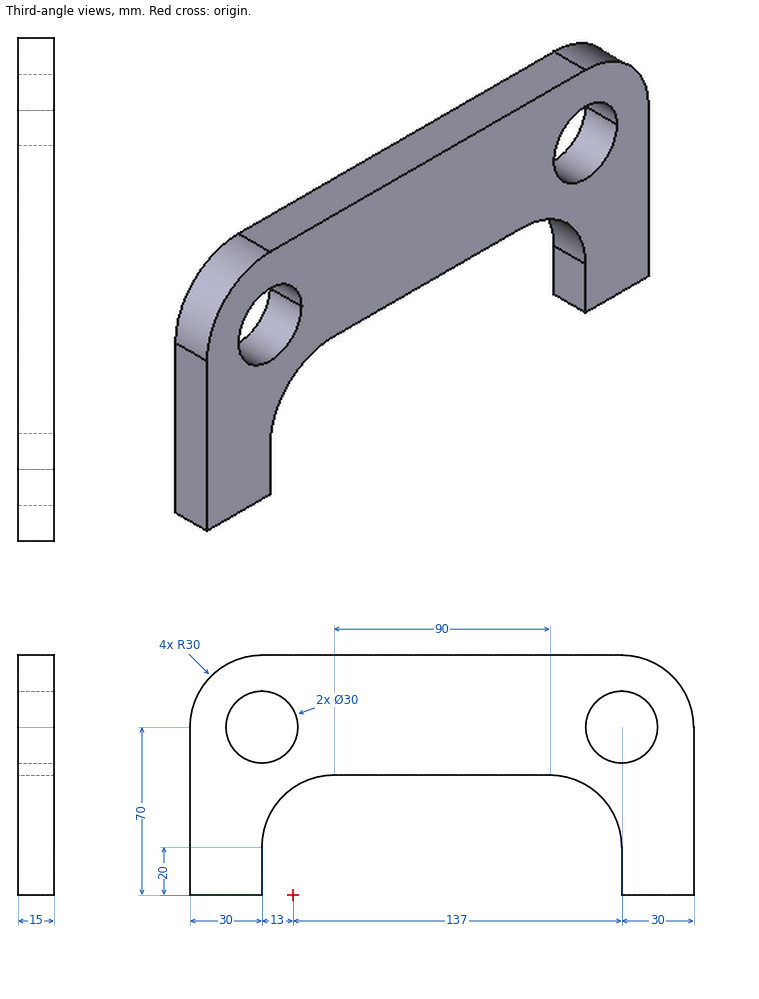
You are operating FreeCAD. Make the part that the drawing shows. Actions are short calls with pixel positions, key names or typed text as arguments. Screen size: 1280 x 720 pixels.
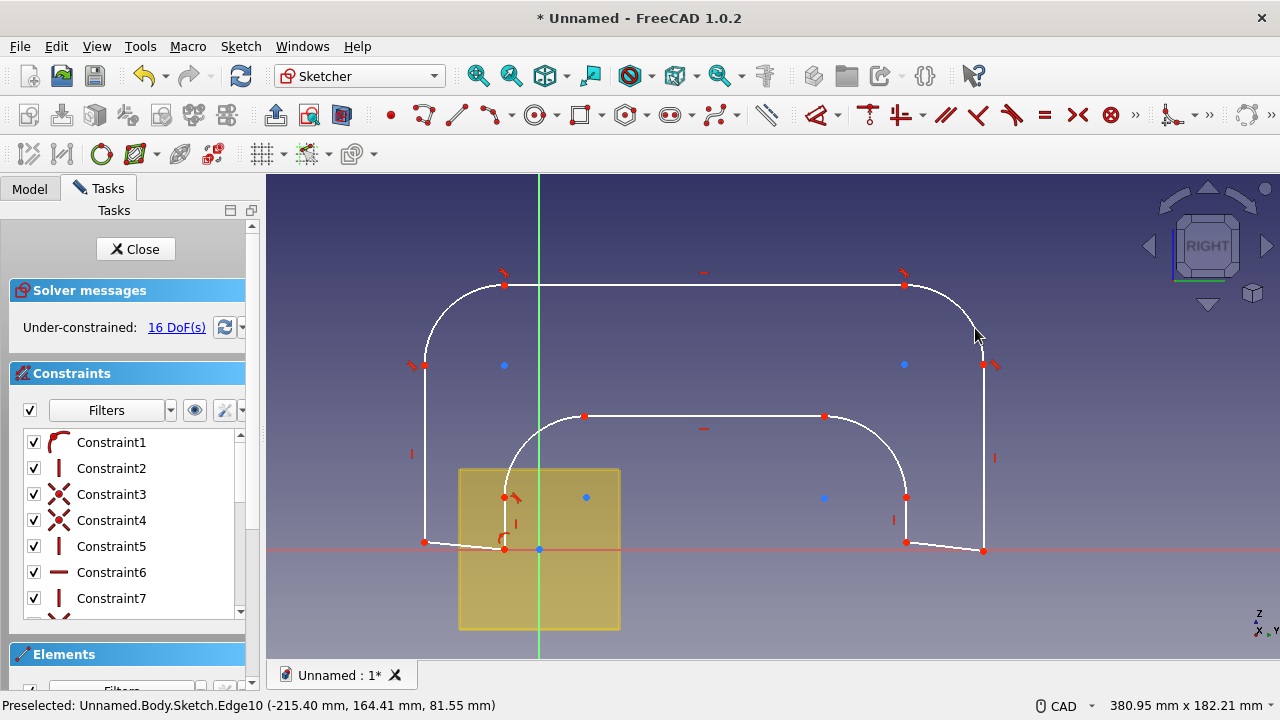
click(906, 529)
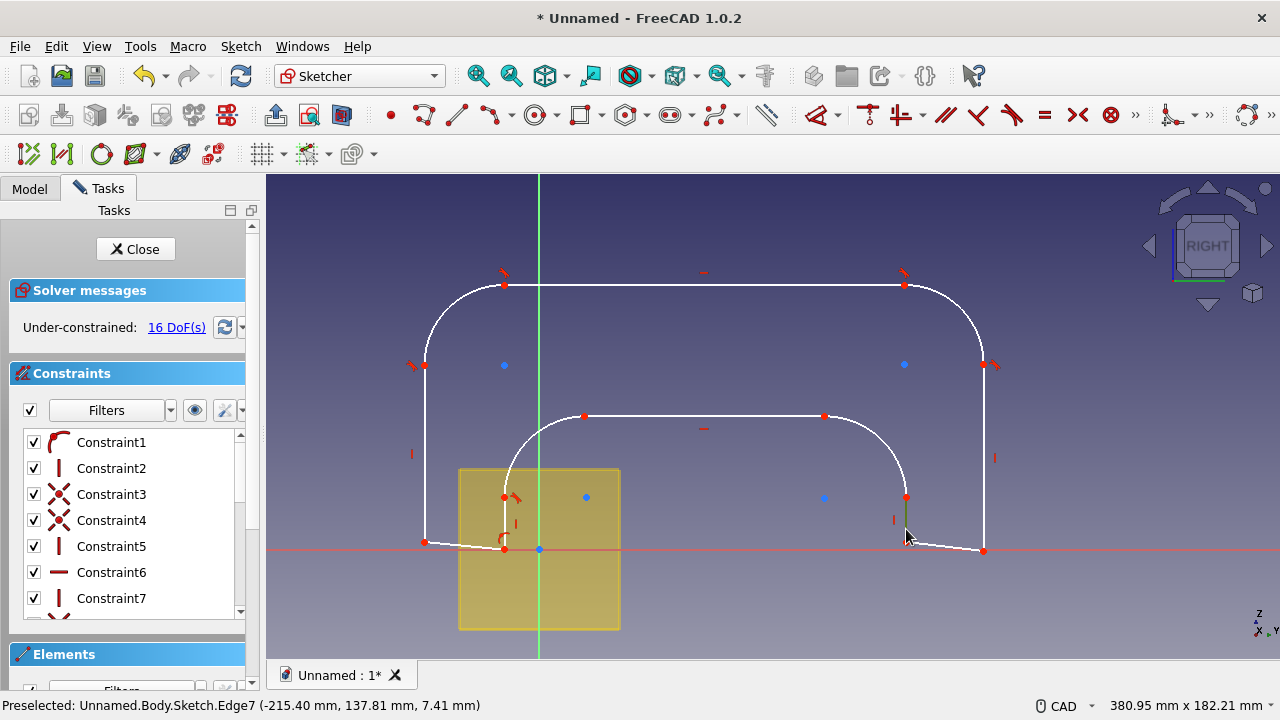
click(897, 460)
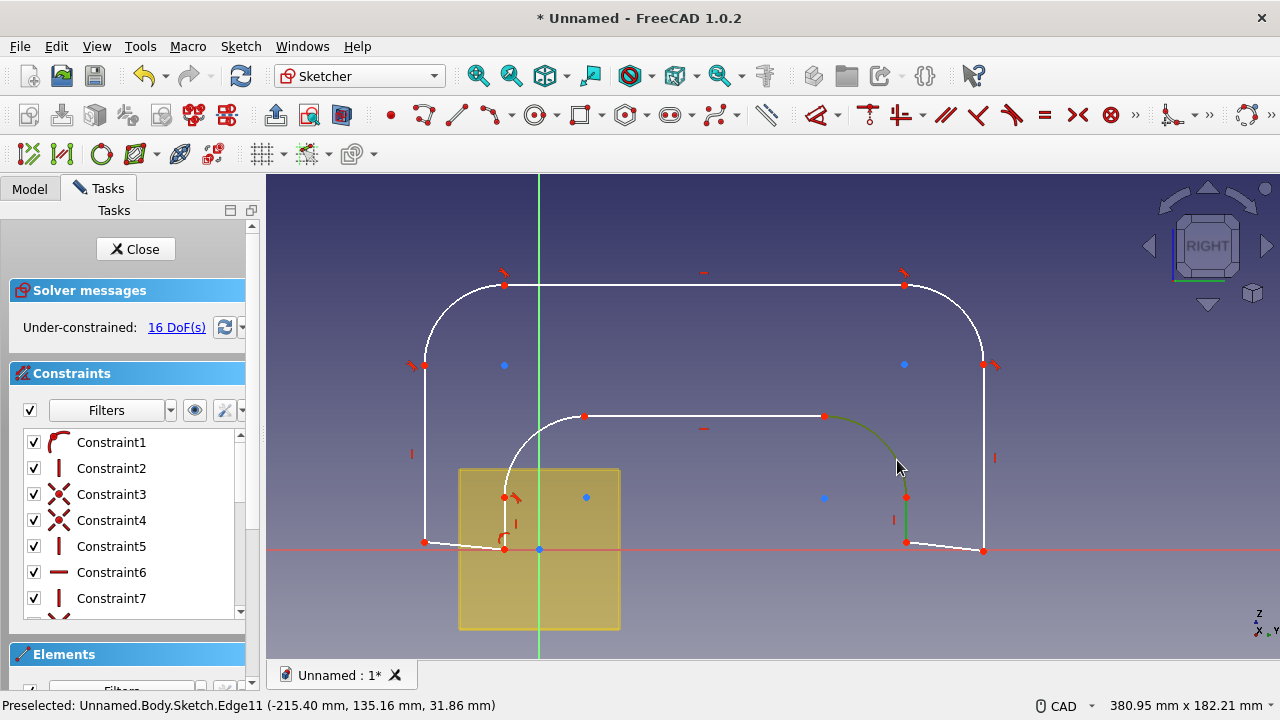
key(t)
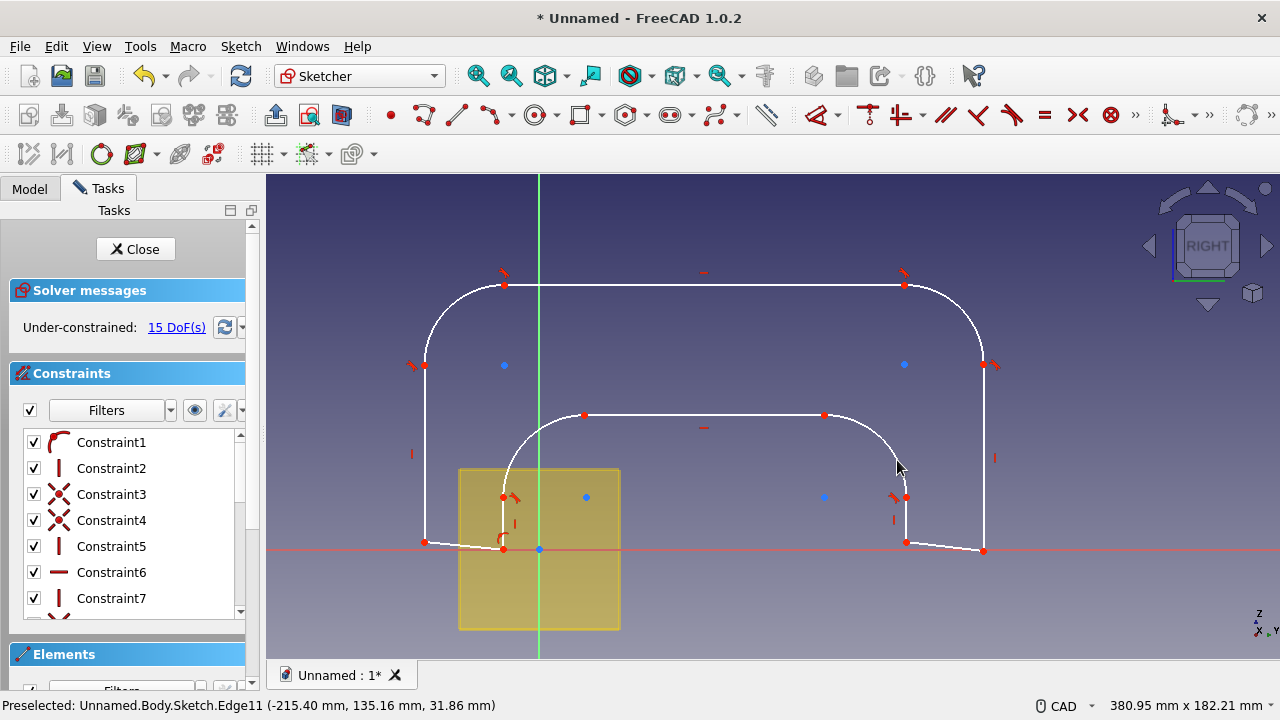
click(753, 415)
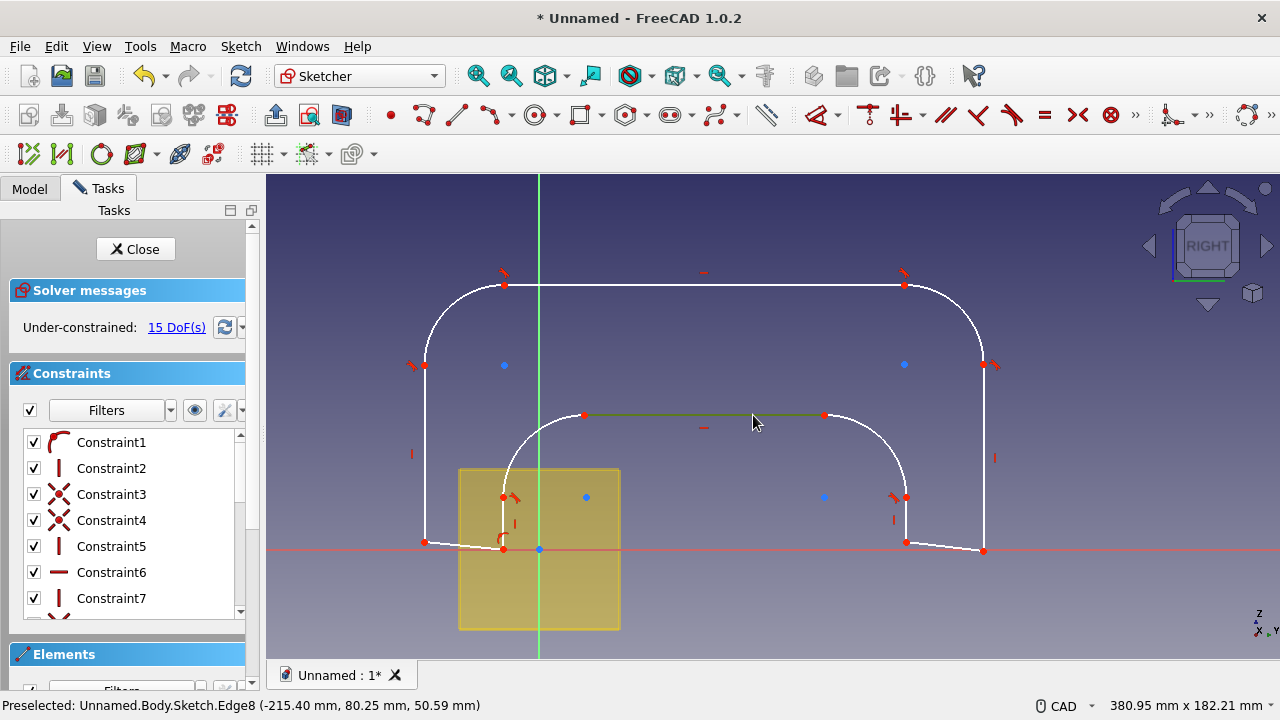
click(897, 460)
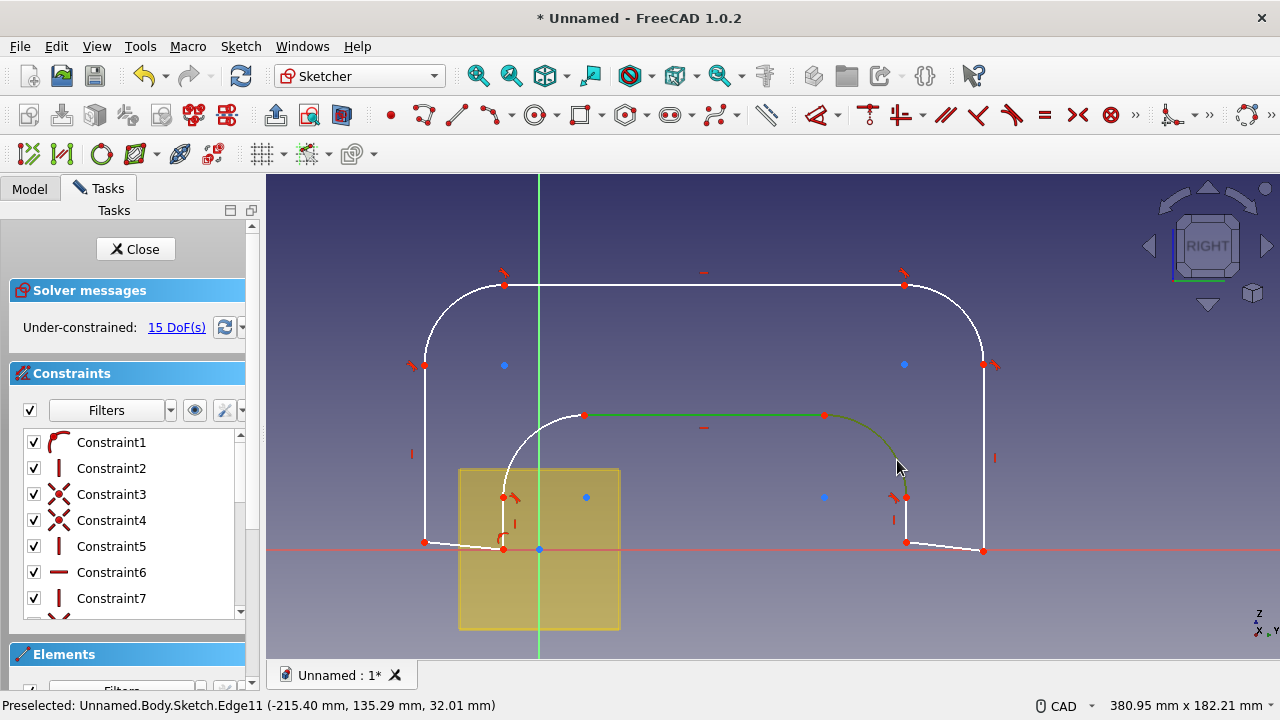
key(t)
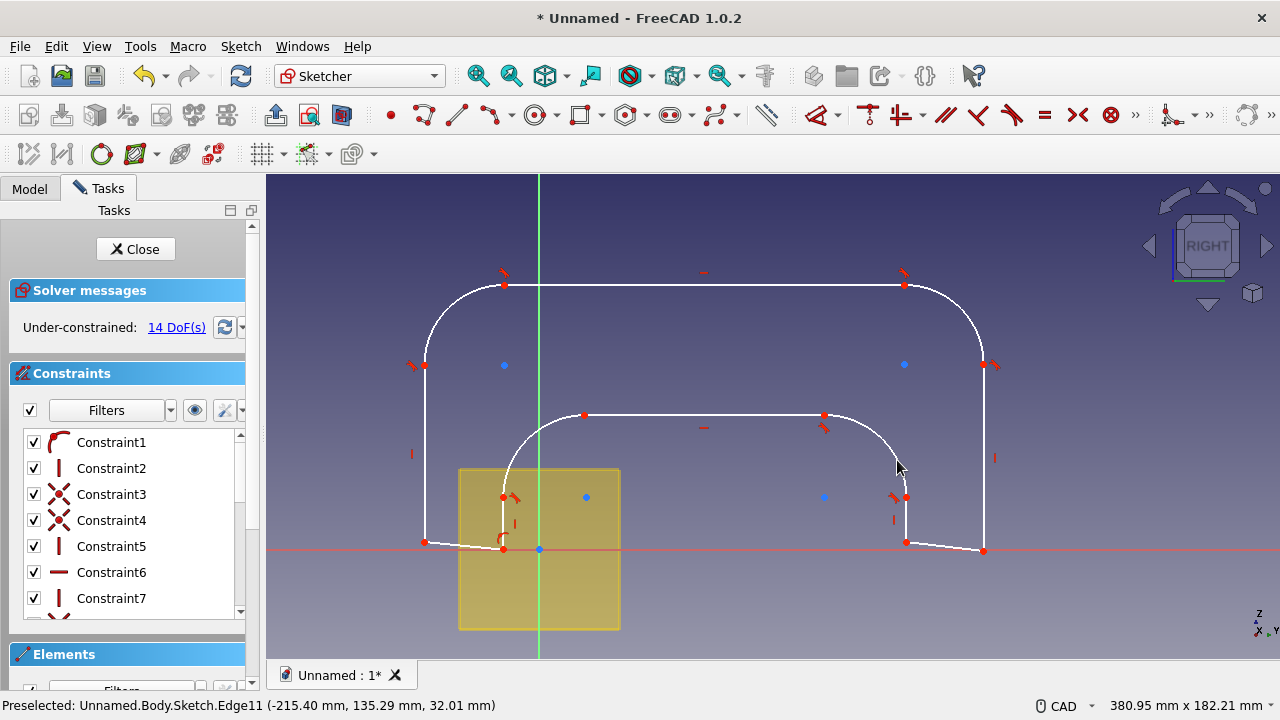
click(752, 415)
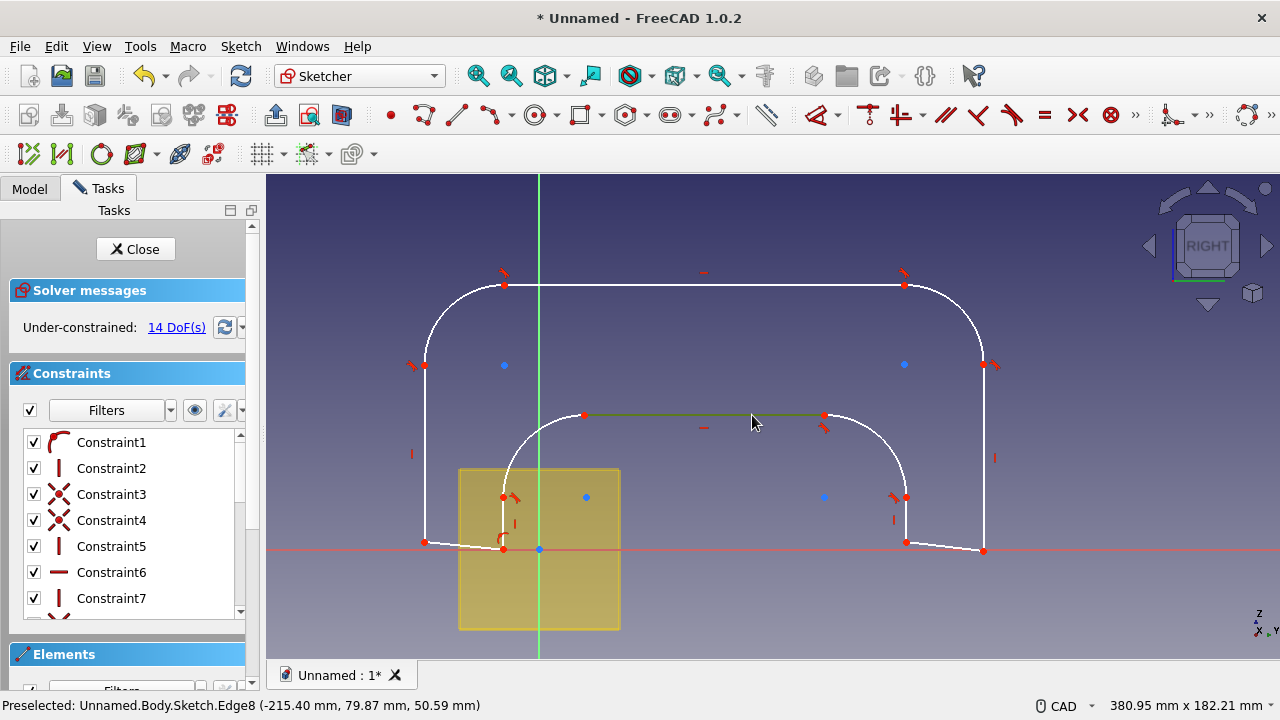
click(512, 461)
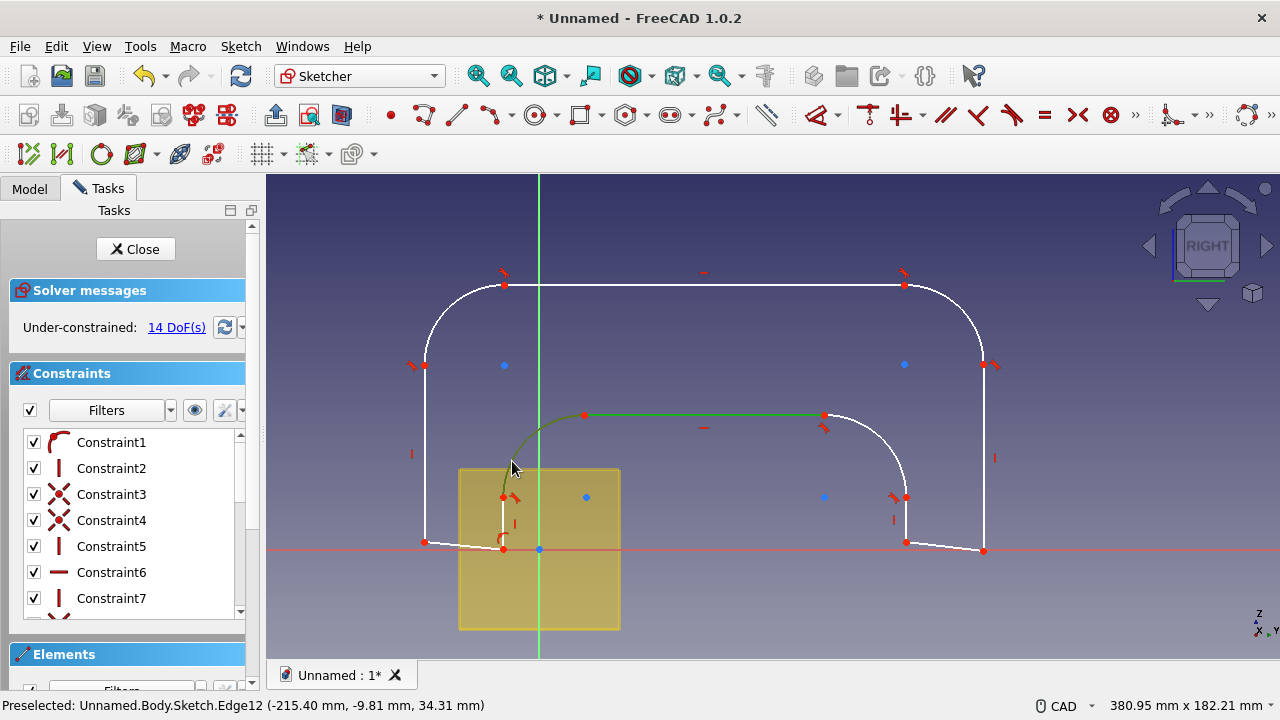
key(t)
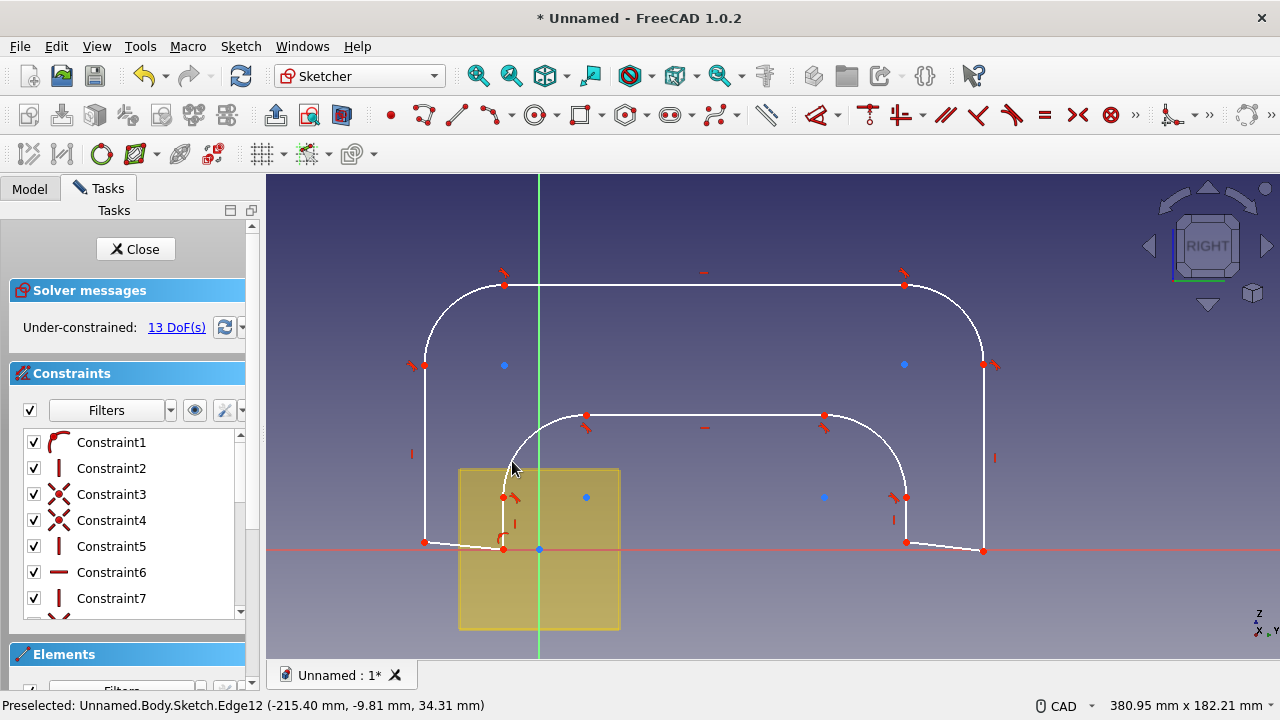
click(480, 547)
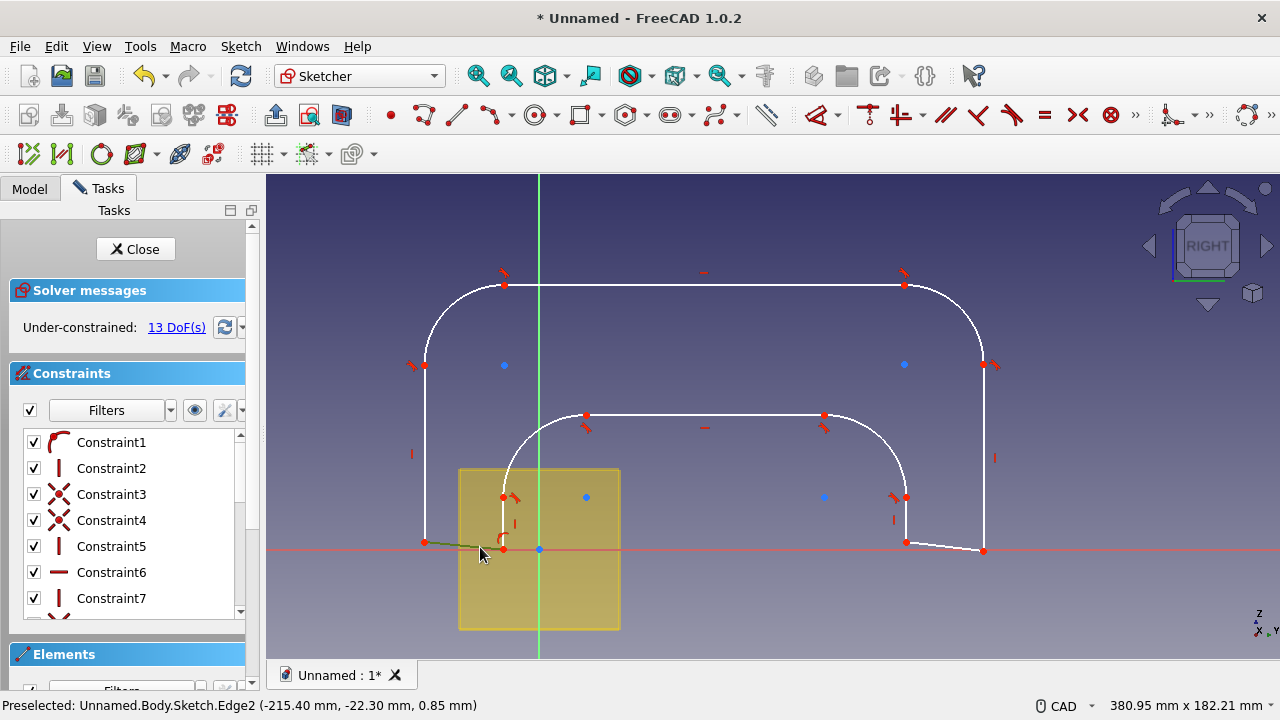
key(h)